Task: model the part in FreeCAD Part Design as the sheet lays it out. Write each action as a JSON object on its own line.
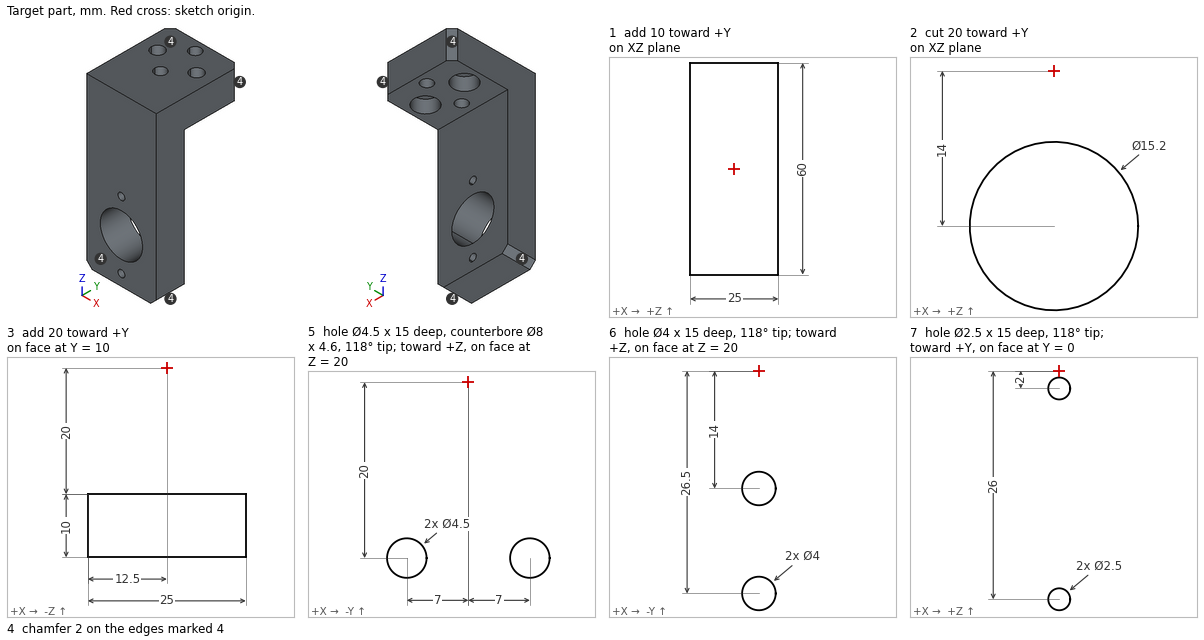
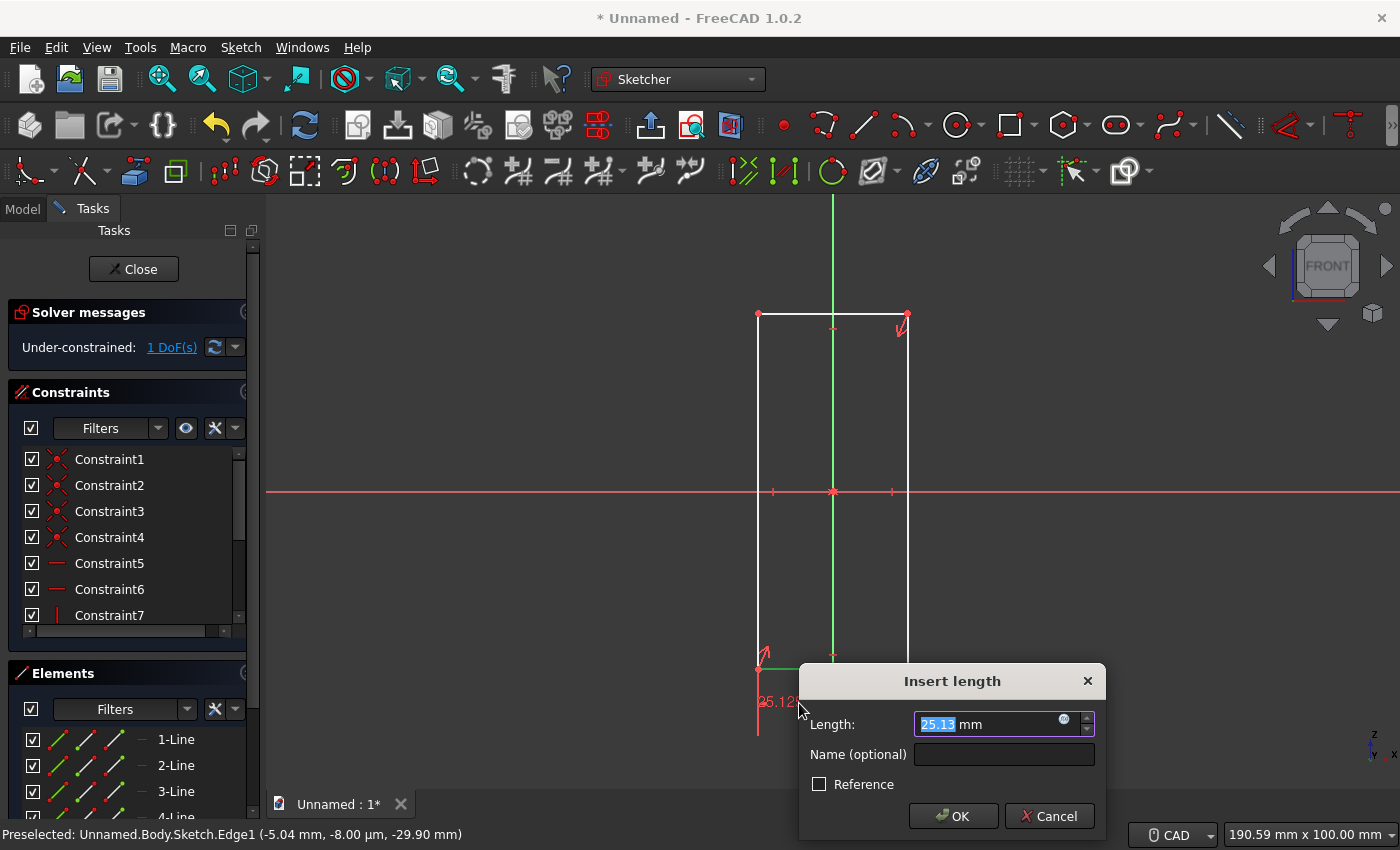
{"action": "type", "text": "25"}
{"action": "key", "text": "Return"}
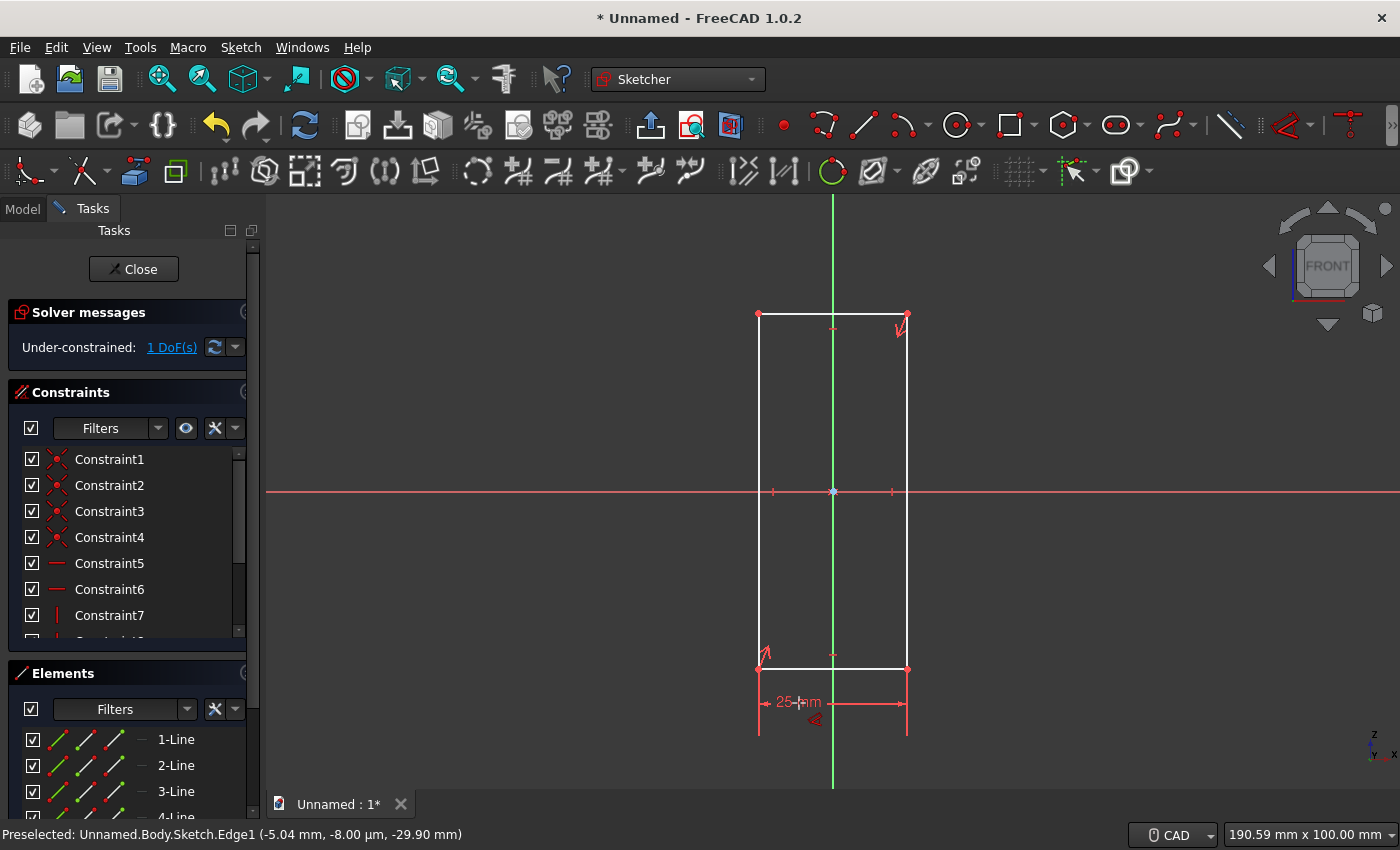
{"action": "left_click", "coordinate": [907, 563]}
{"action": "left_click", "coordinate": [941, 410]}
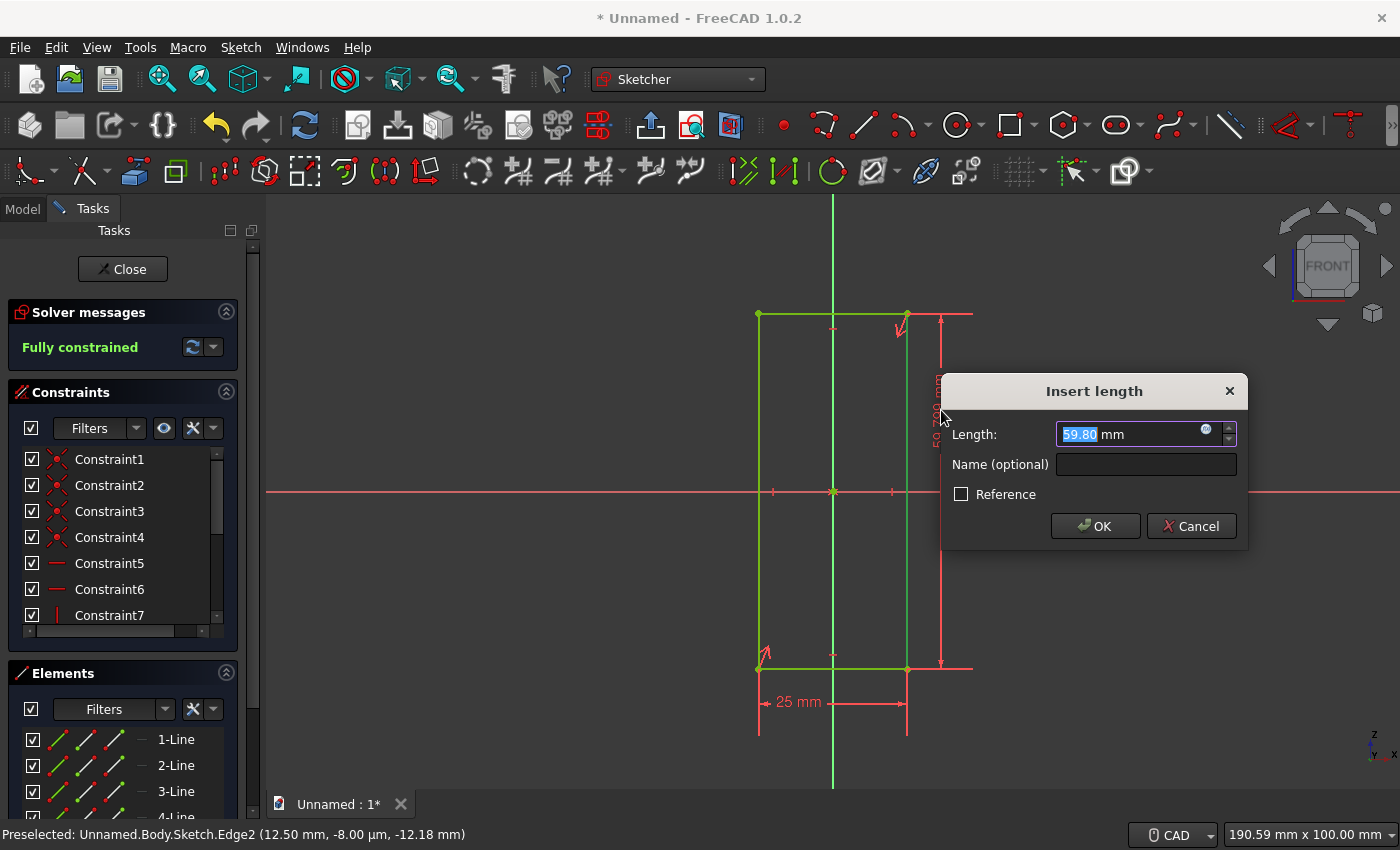
{"action": "type", "text": "60"}
{"action": "key", "text": "Return"}
{"action": "key", "text": "Escape"}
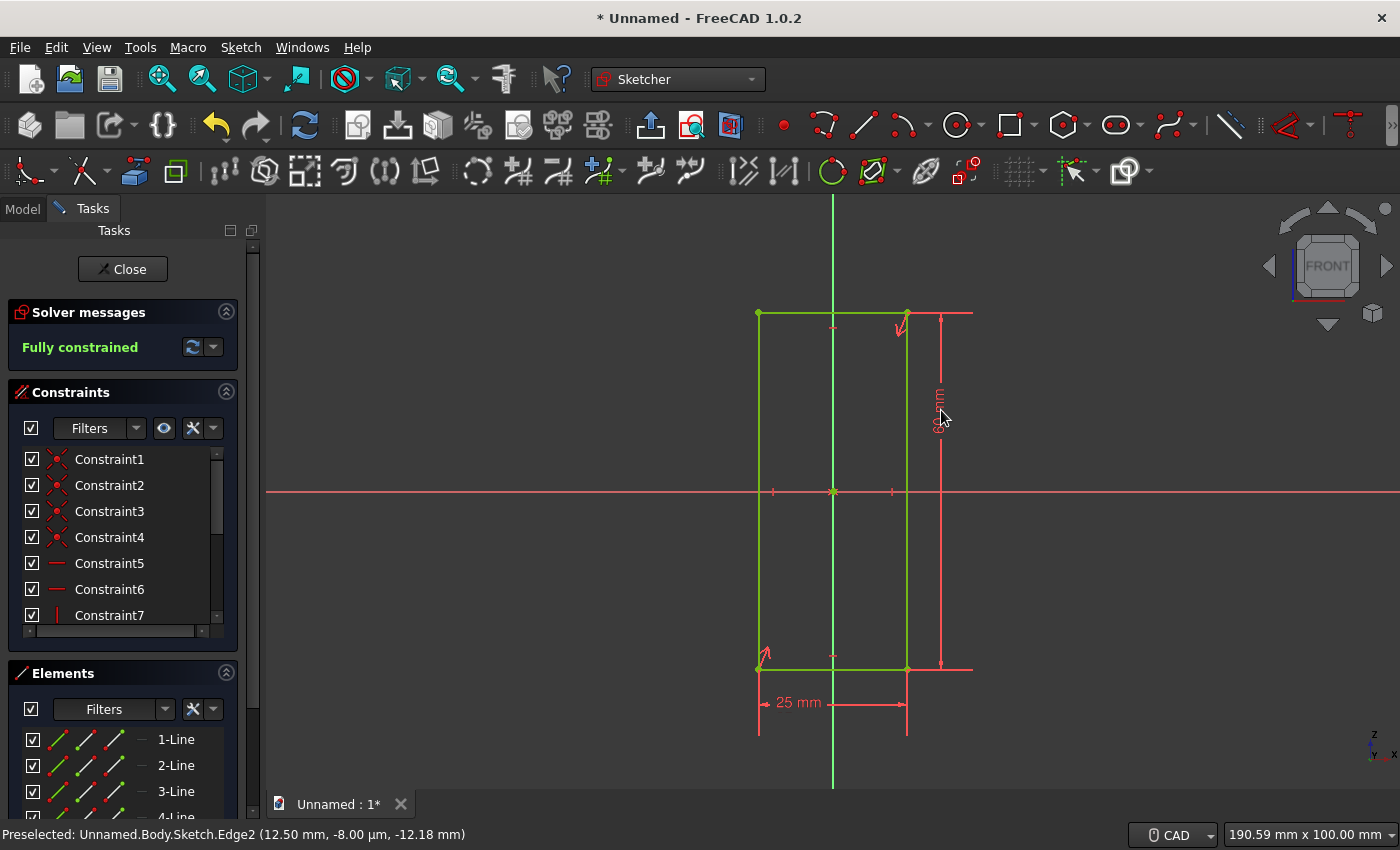
{"action": "left_click", "coordinate": [123, 269]}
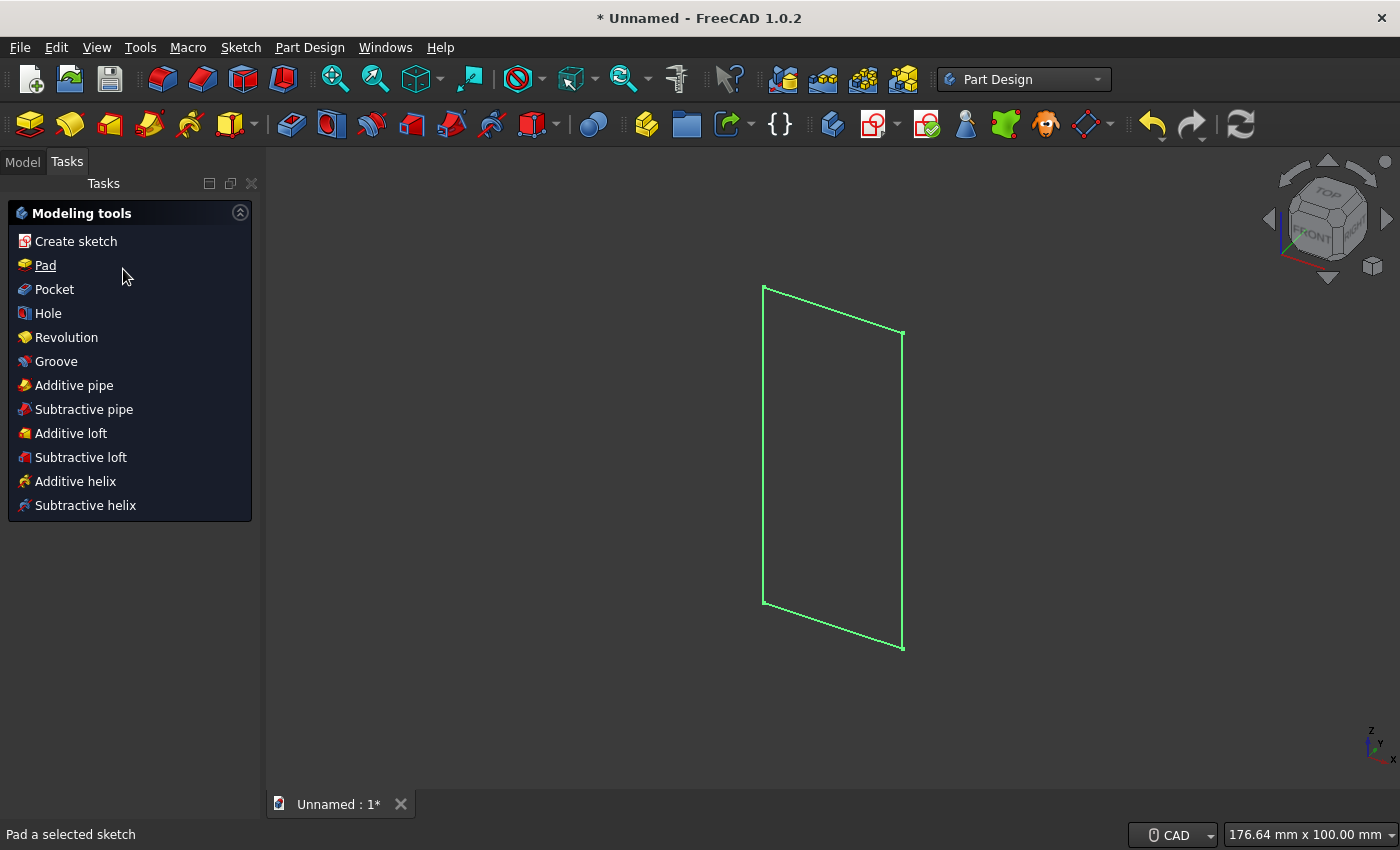
{"action": "left_click", "coordinate": [30, 124]}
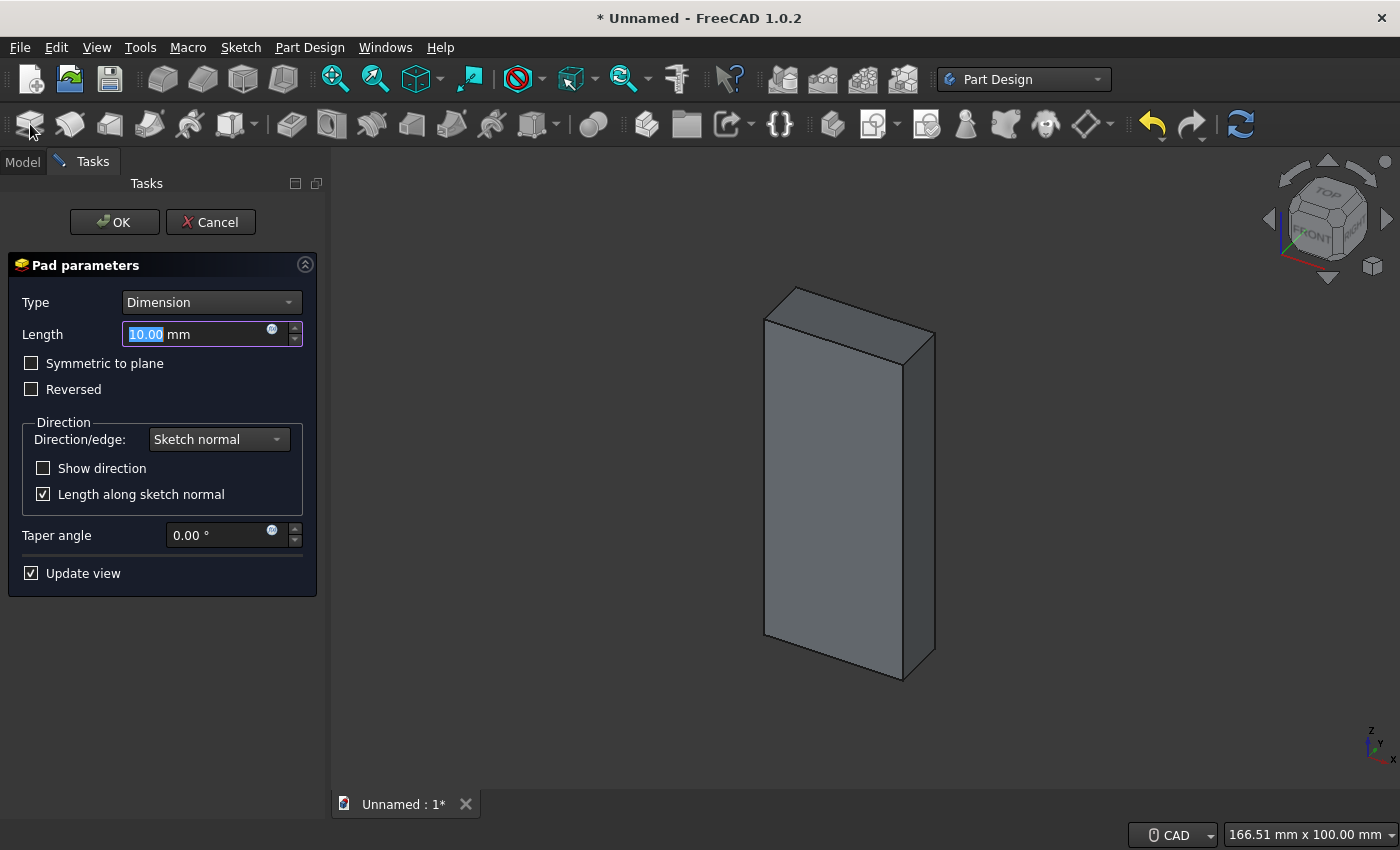
{"action": "type", "text": "10"}
{"action": "key", "text": "Tab"}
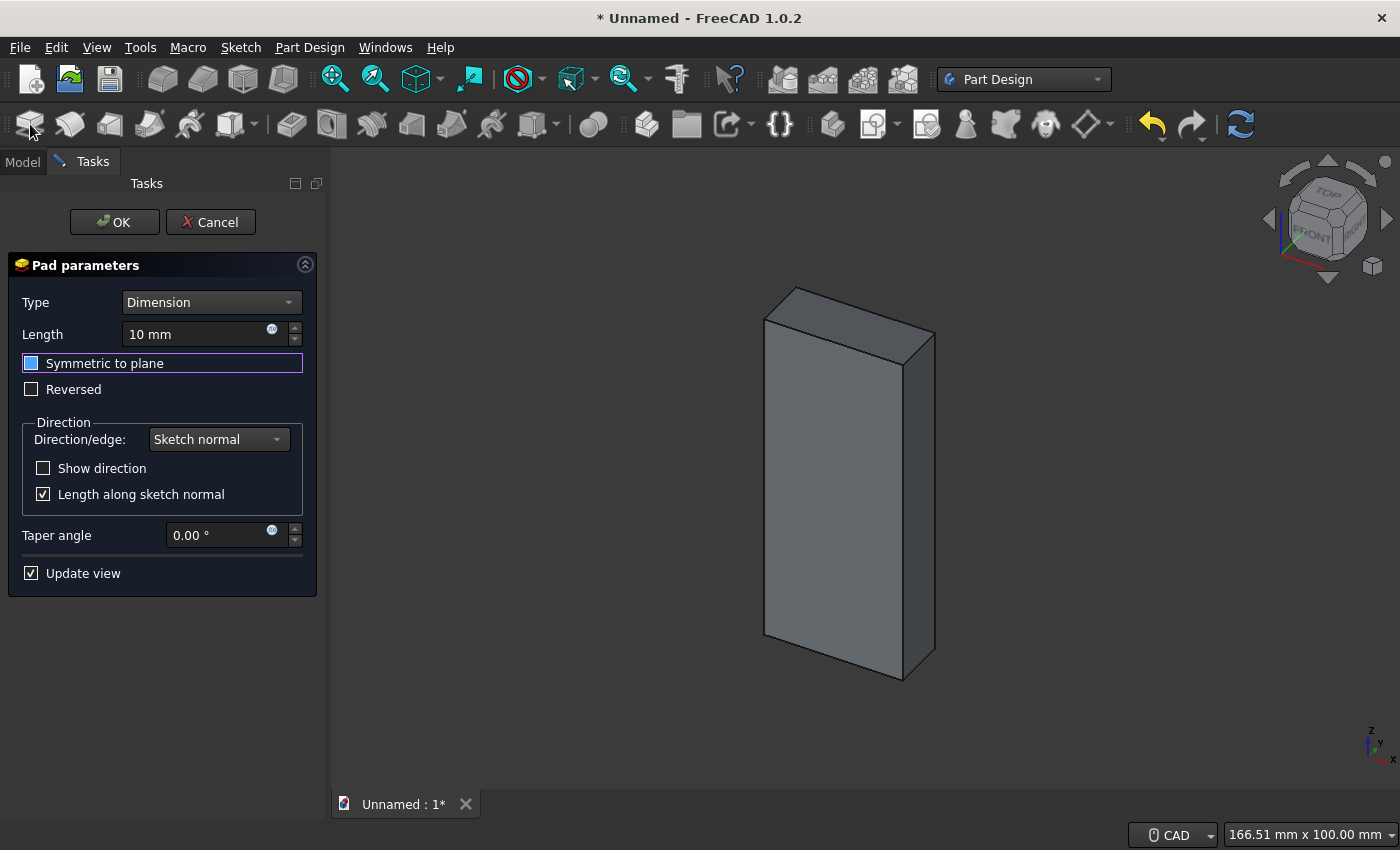
{"action": "left_click", "coordinate": [30, 389]}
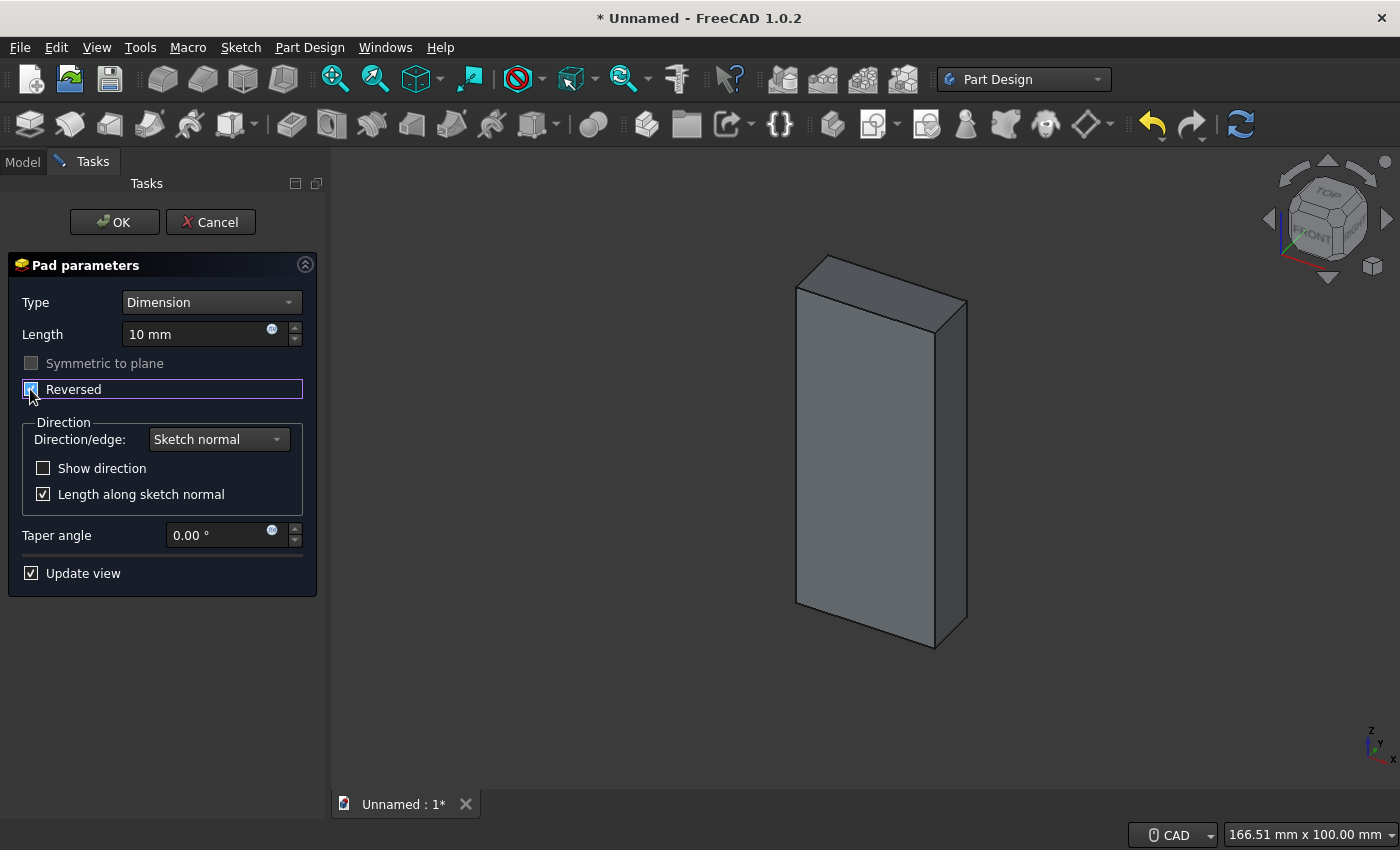
{"action": "left_click", "coordinate": [115, 222]}